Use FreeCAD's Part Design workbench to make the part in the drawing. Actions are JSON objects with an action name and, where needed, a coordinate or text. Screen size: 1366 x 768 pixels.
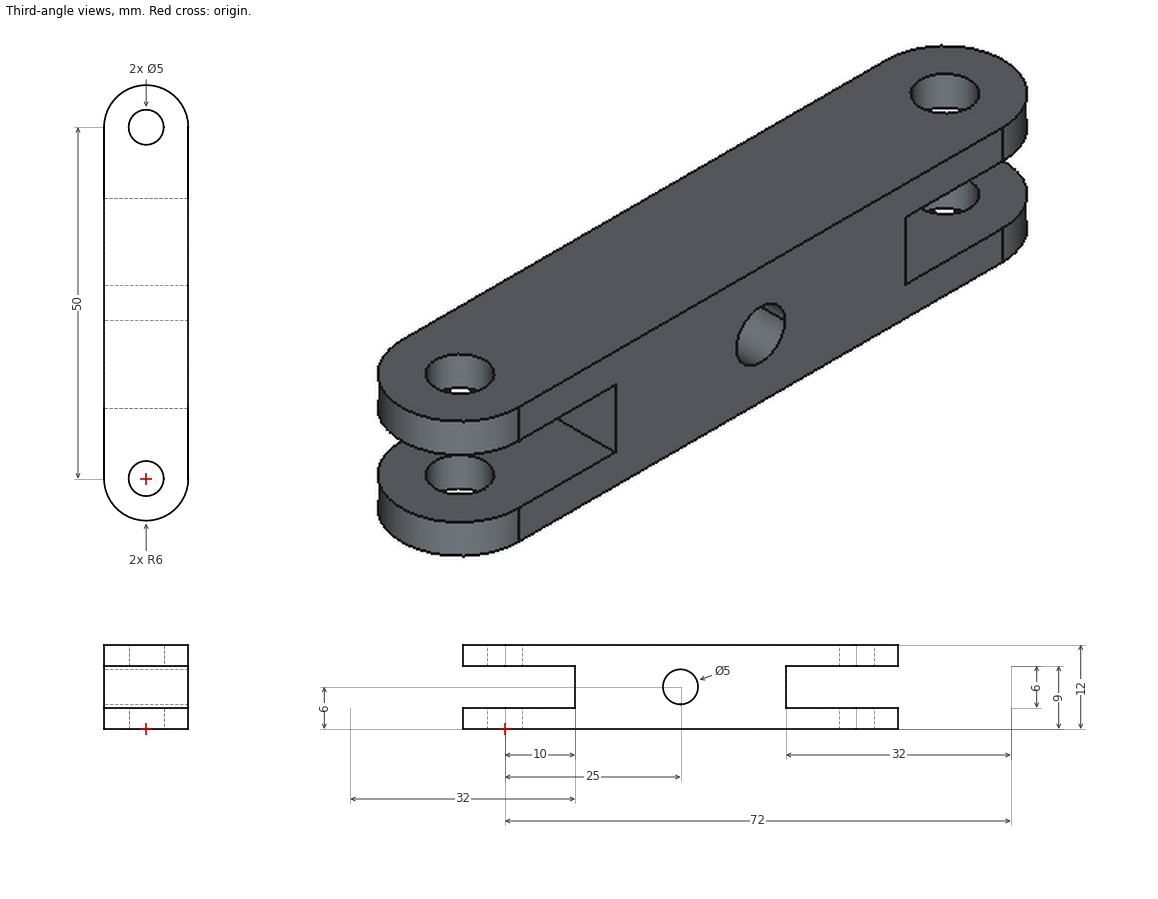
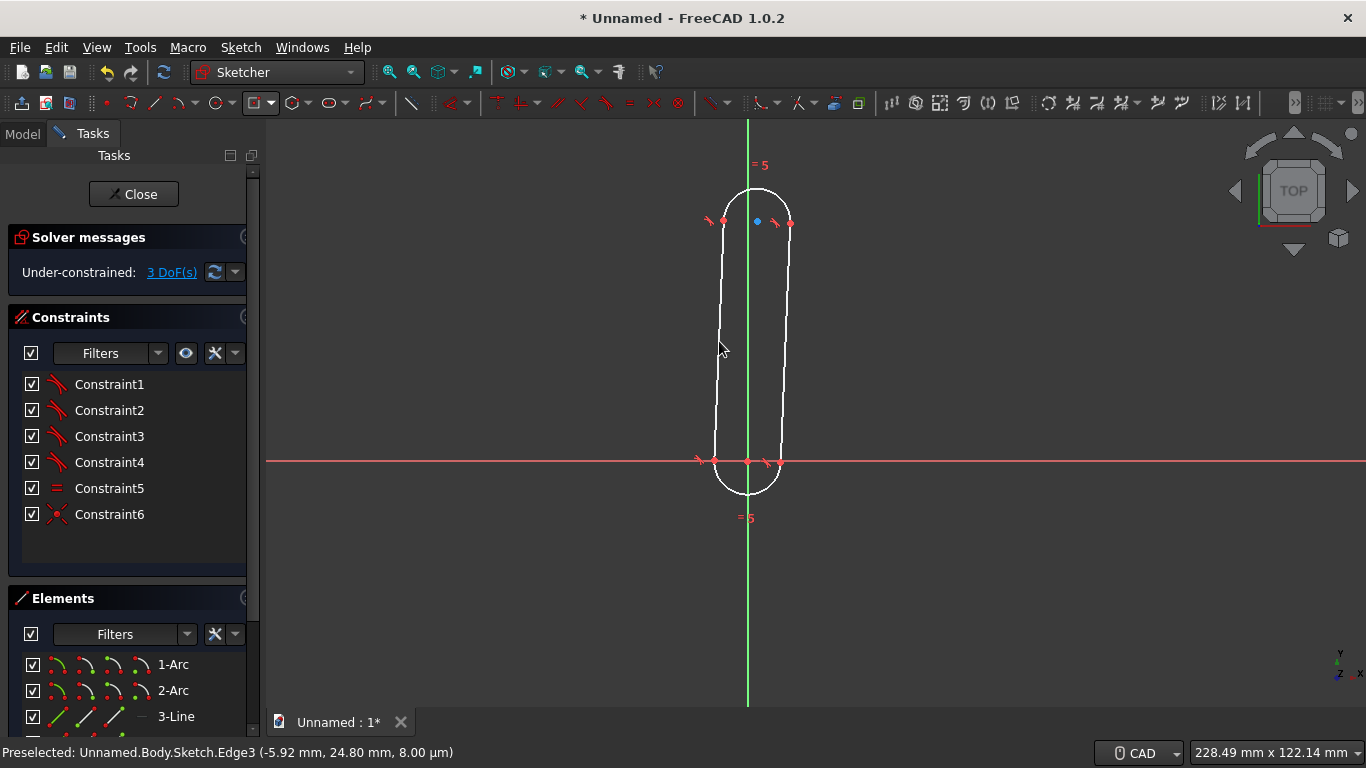
{"action": "left_click", "coordinate": [717, 388]}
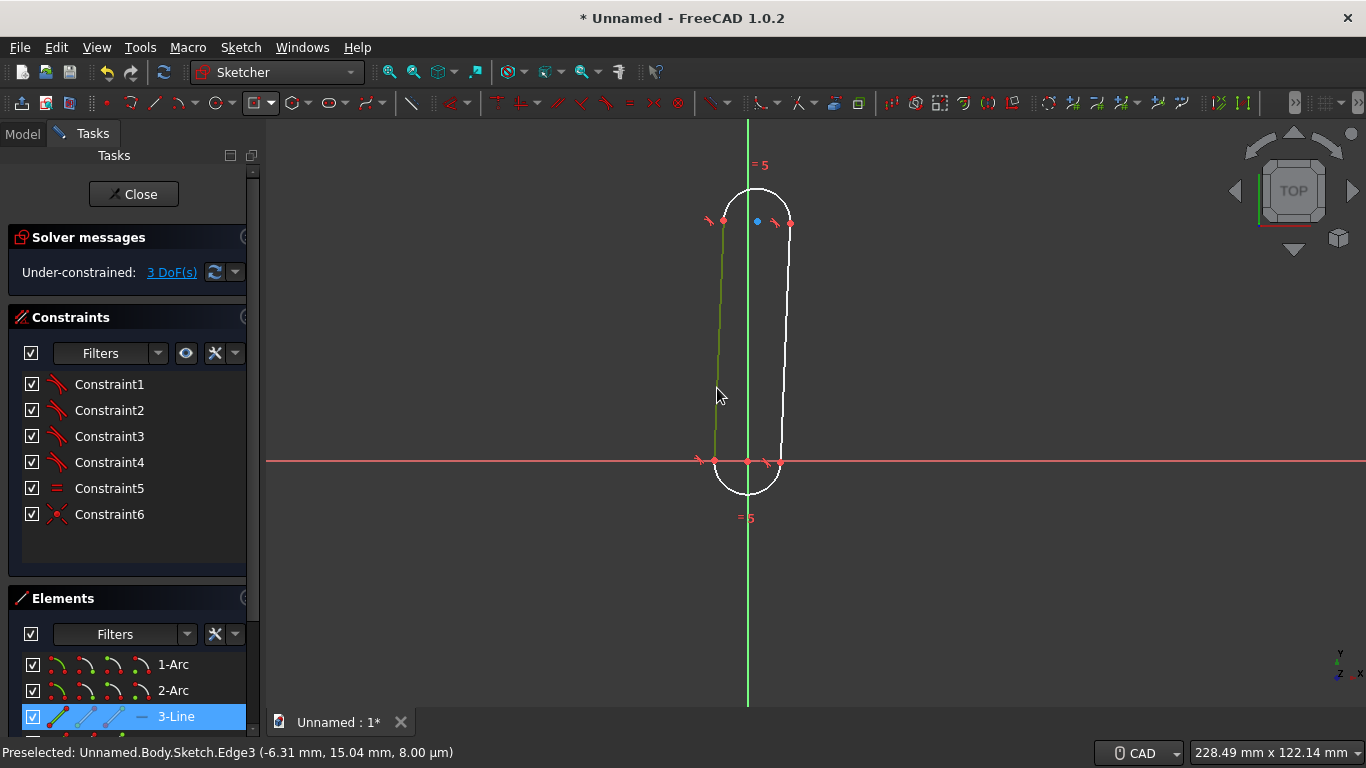
{"action": "key", "text": "v"}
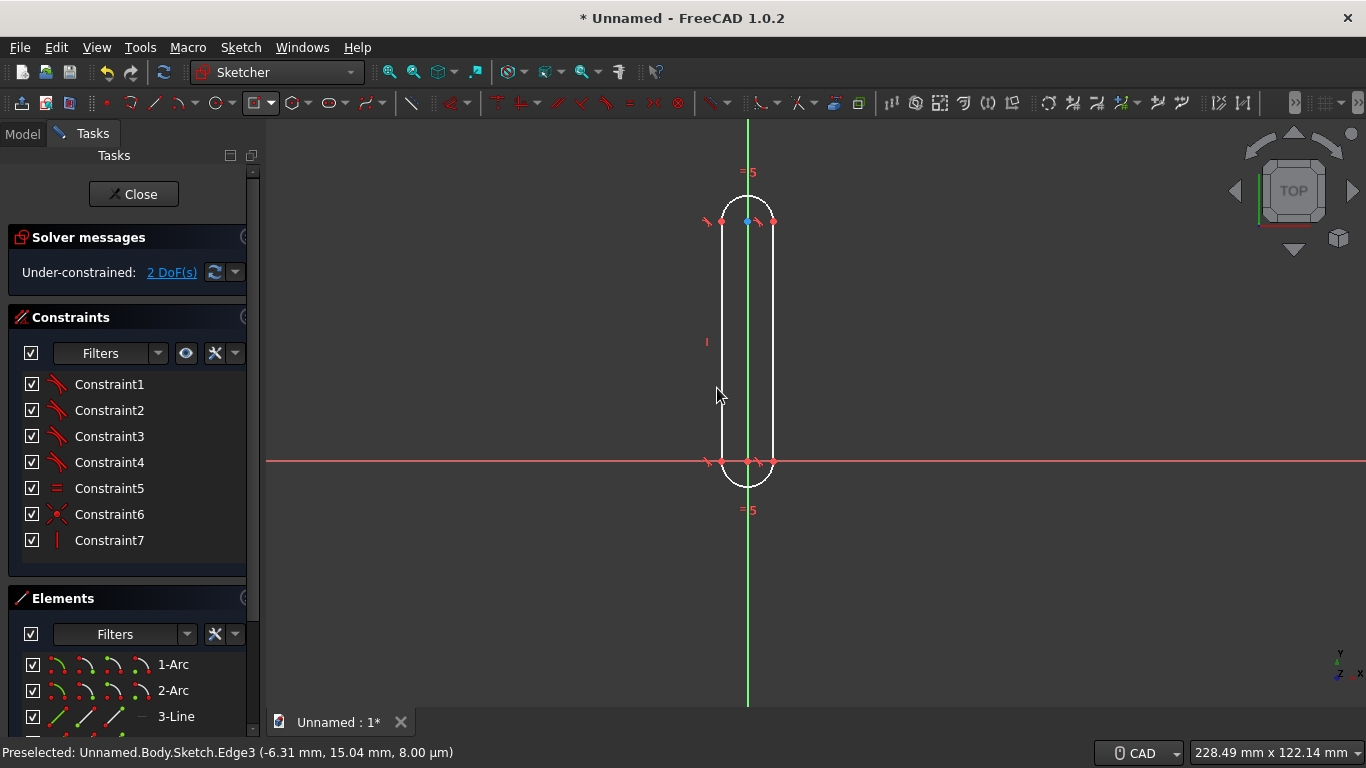
{"action": "scroll", "coordinate": [732, 482], "scroll_direction": "up", "scroll_amount": 2}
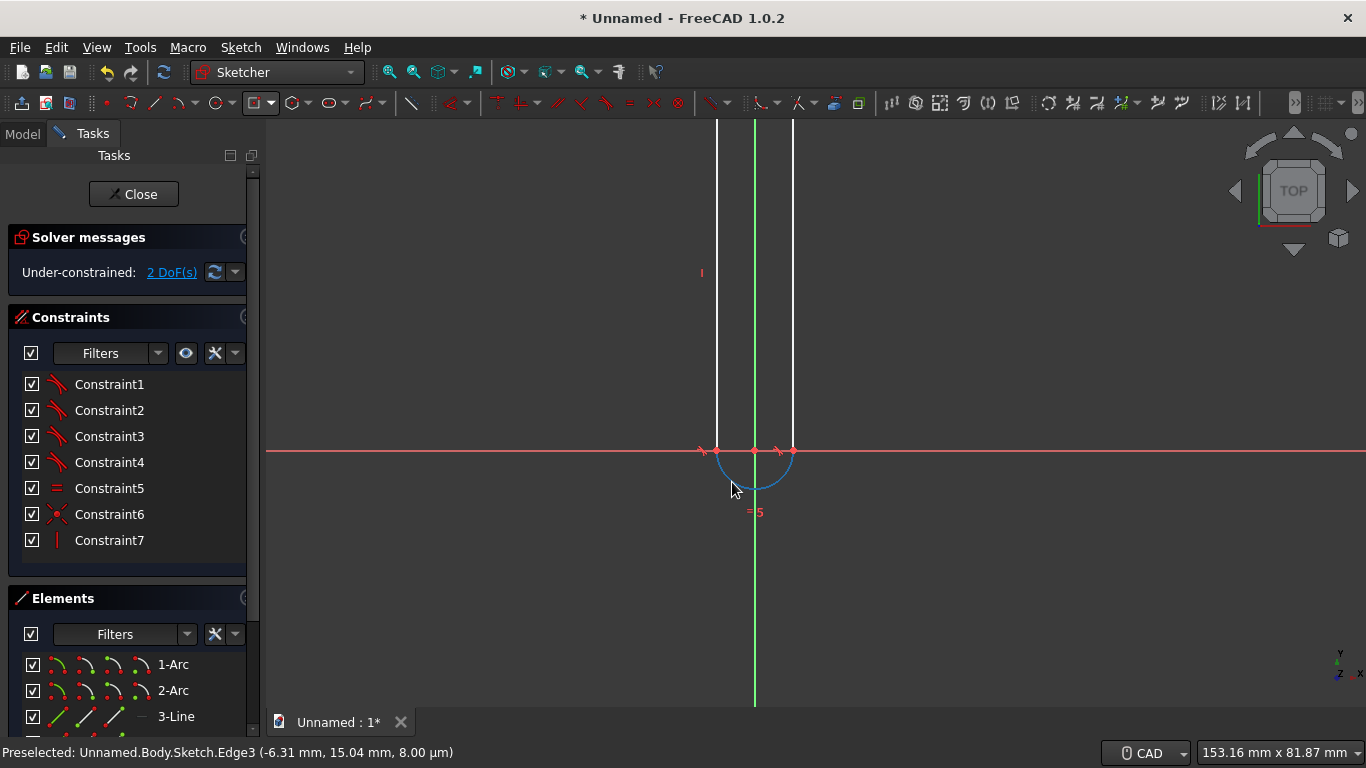
{"action": "left_click", "coordinate": [733, 482]}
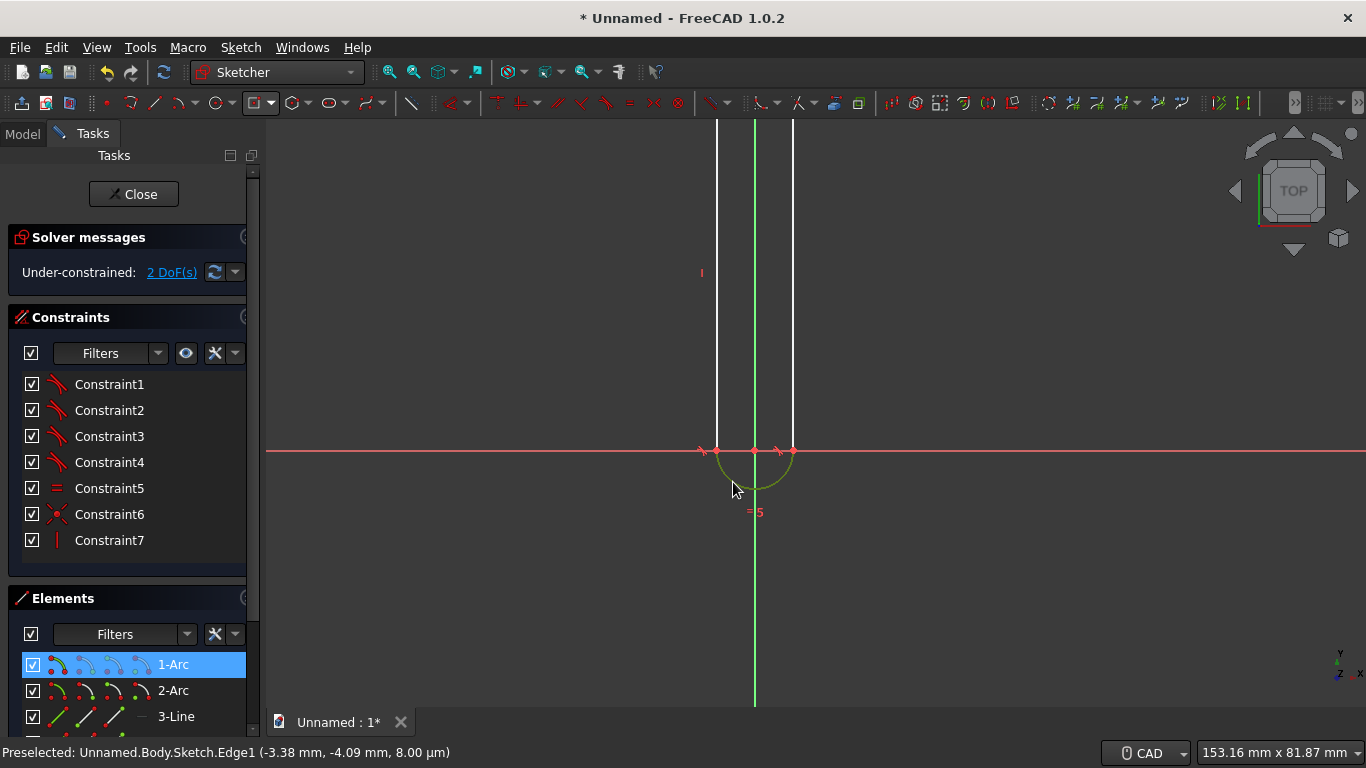
{"action": "left_click", "coordinate": [470, 104]}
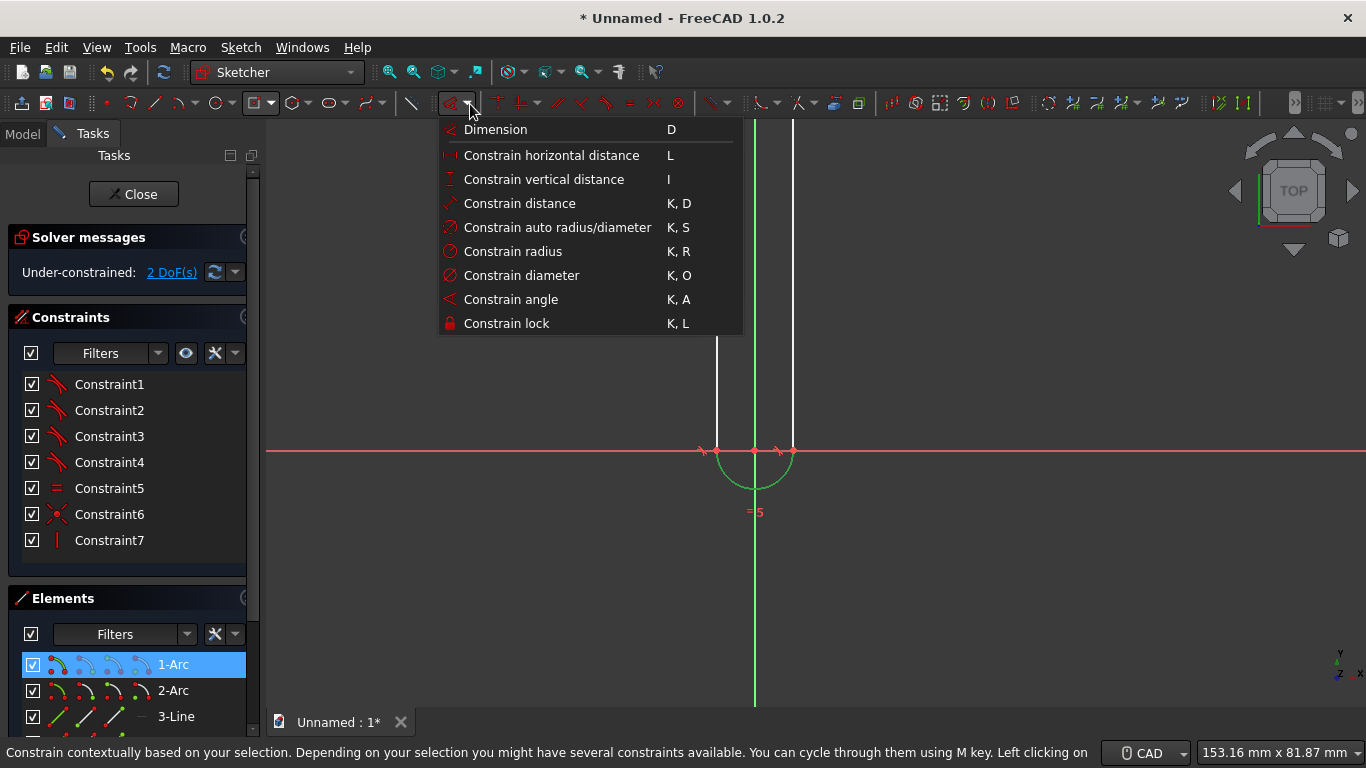
{"action": "left_click", "coordinate": [591, 251]}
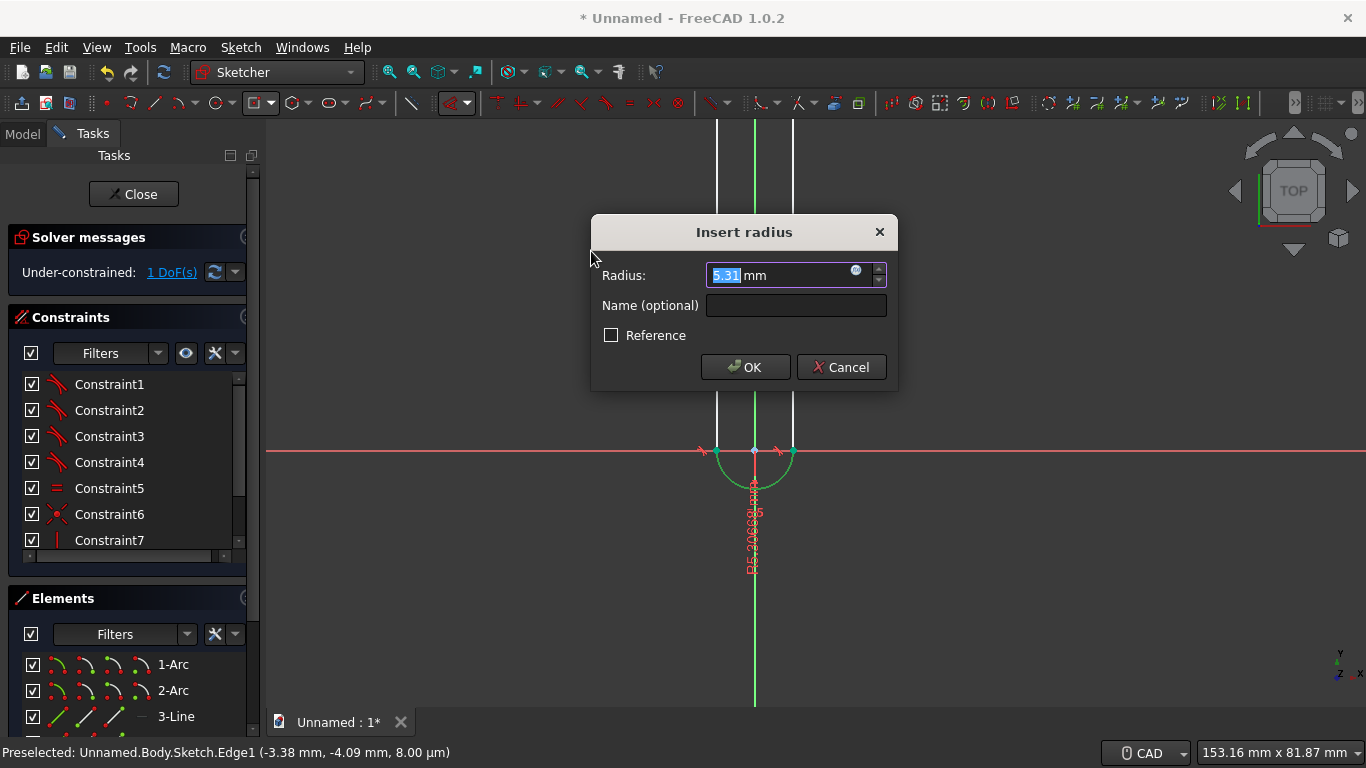
{"action": "type", "text": "6"}
{"action": "key", "text": "Return"}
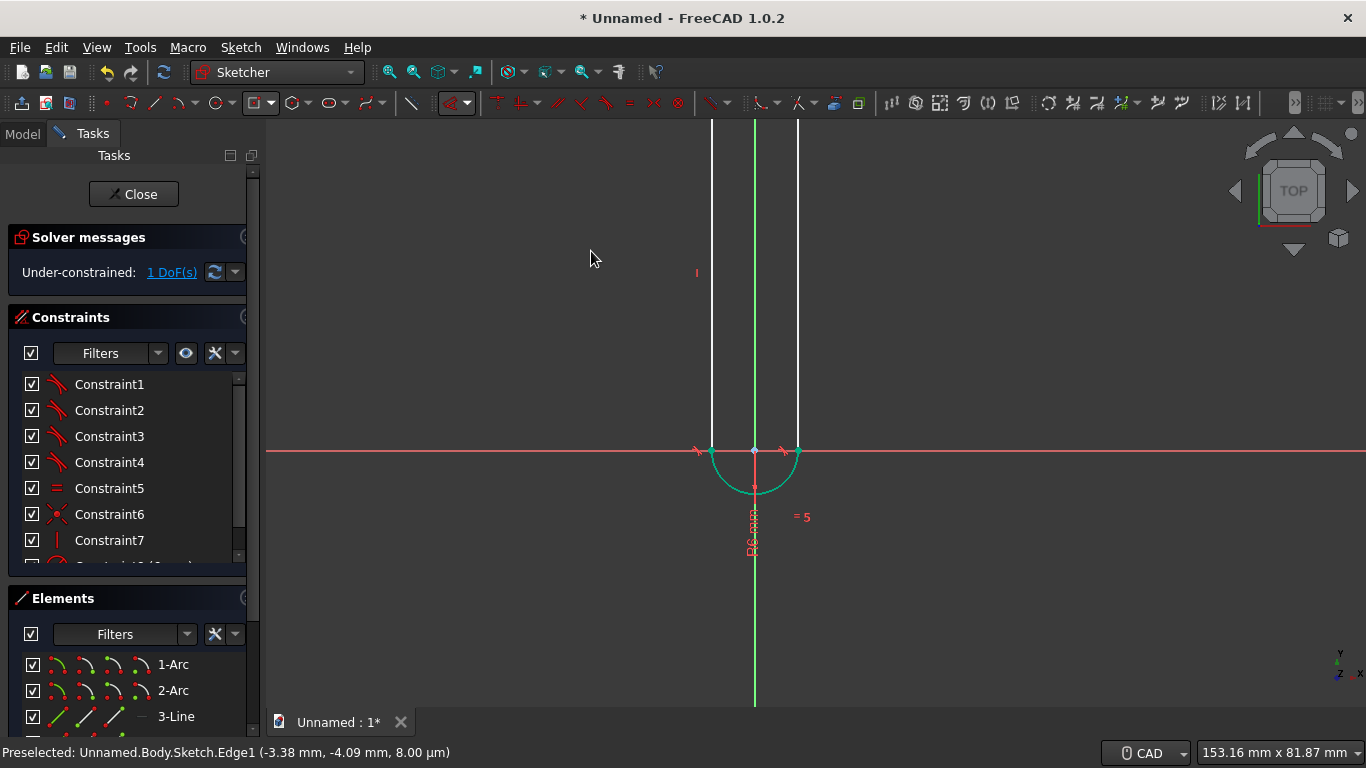
{"action": "left_click", "coordinate": [712, 344]}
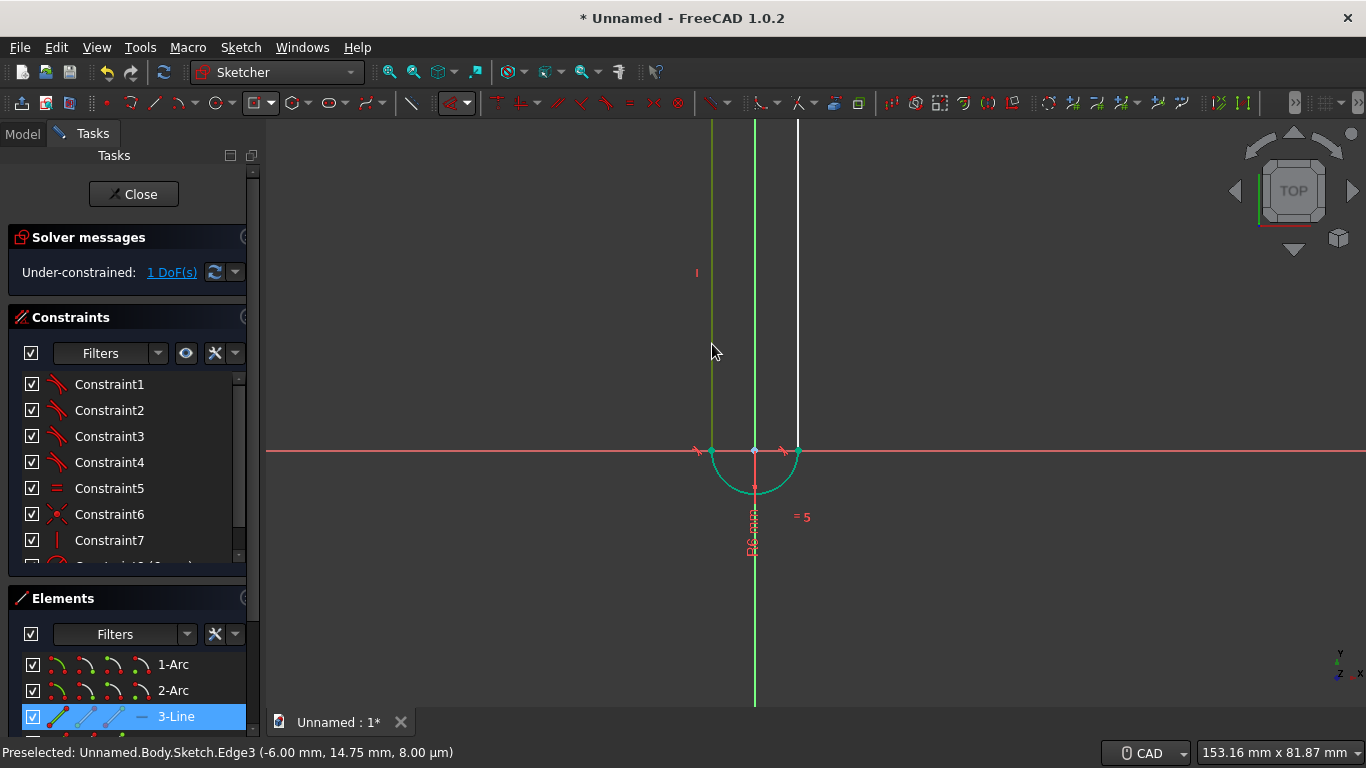
{"action": "key", "text": "i"}